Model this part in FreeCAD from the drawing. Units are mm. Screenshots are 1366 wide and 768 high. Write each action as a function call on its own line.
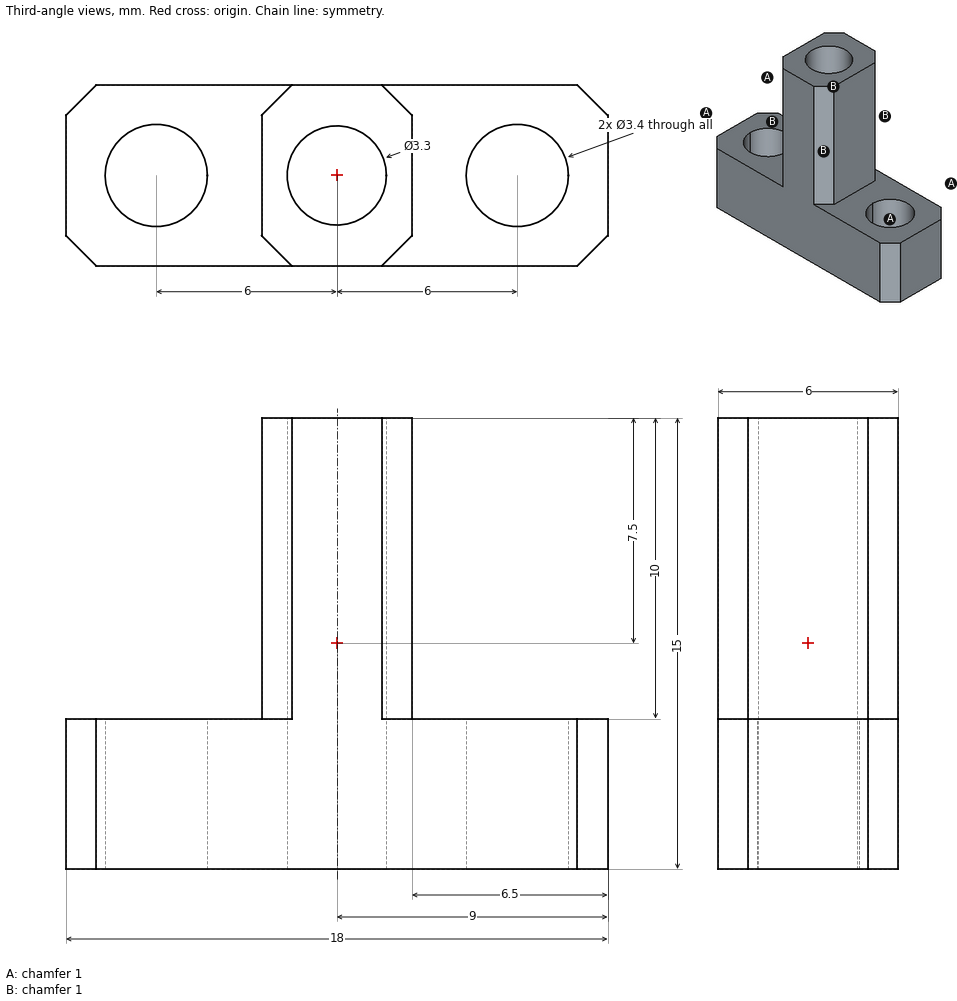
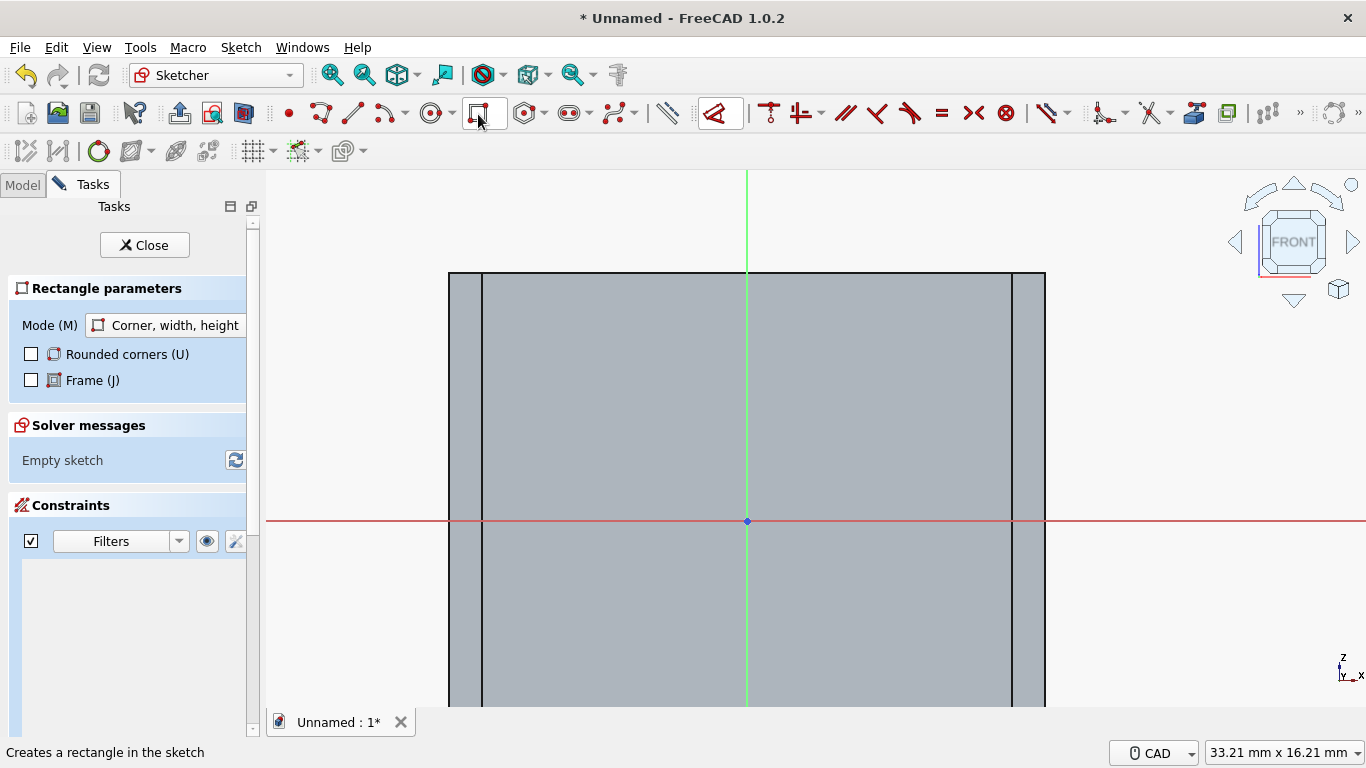
click(830, 273)
click(1045, 604)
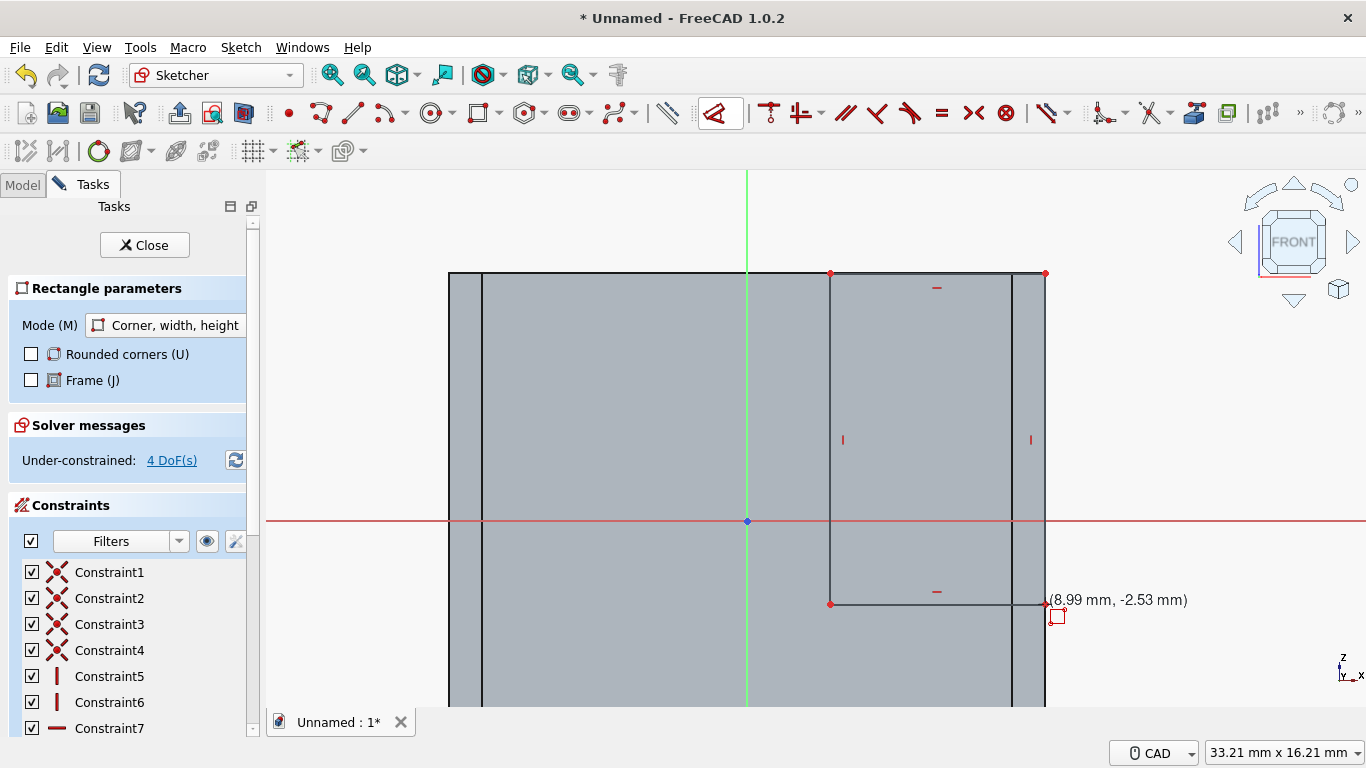
click(449, 273)
click(665, 604)
key(Escape)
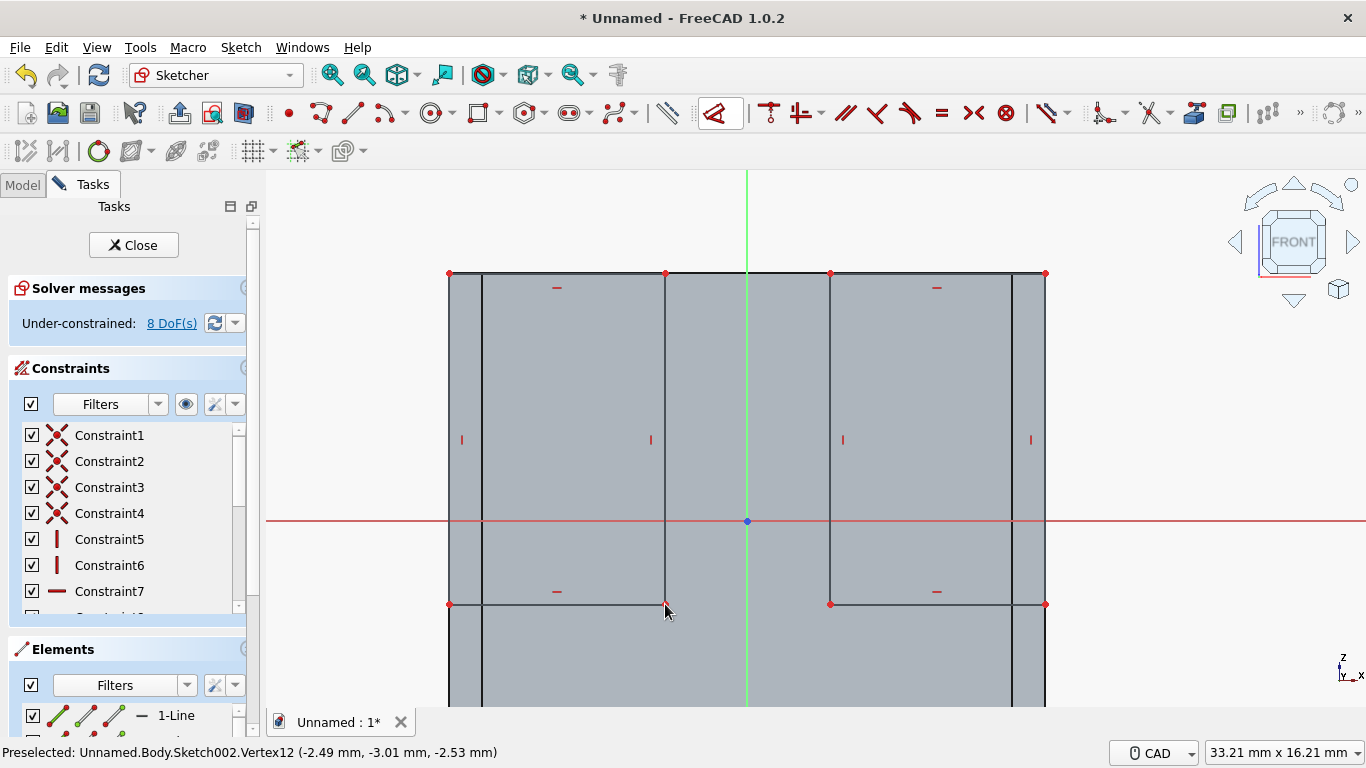
click(1045, 274)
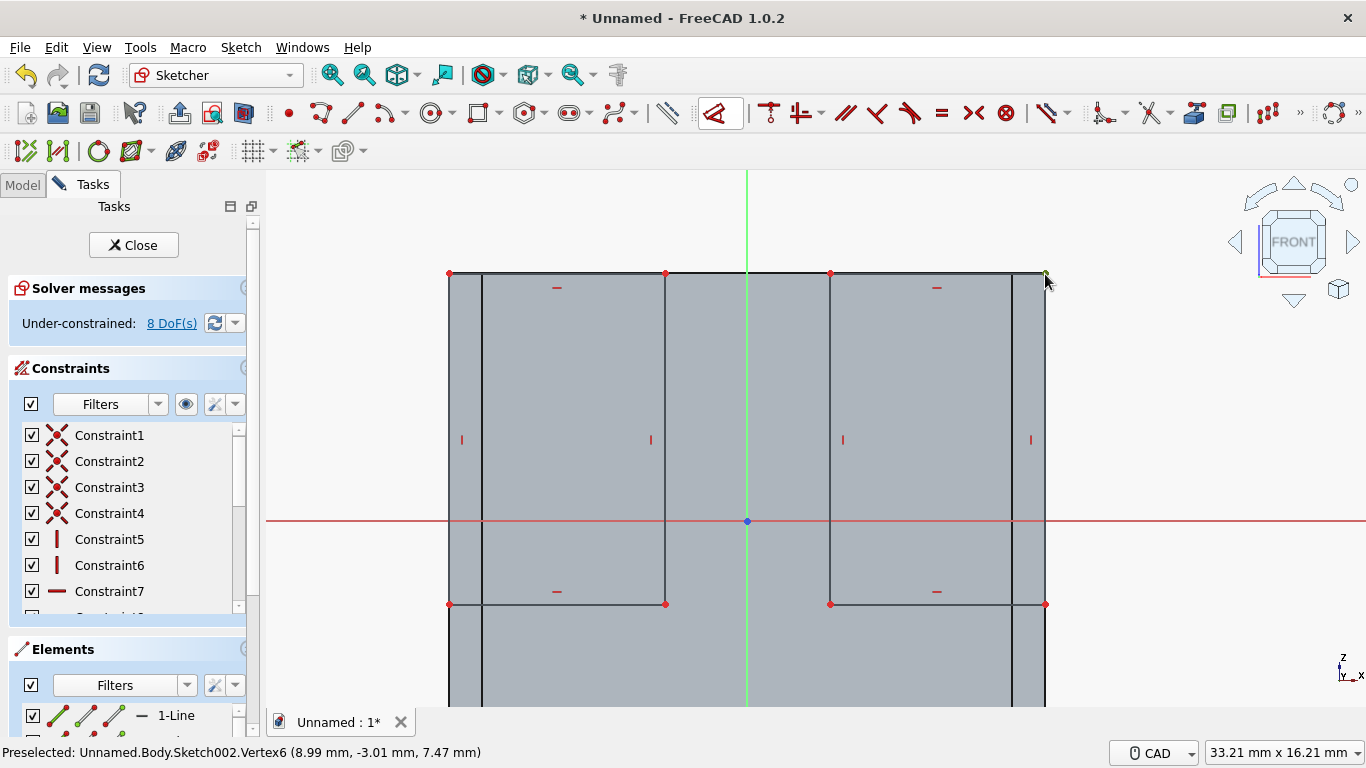
click(449, 274)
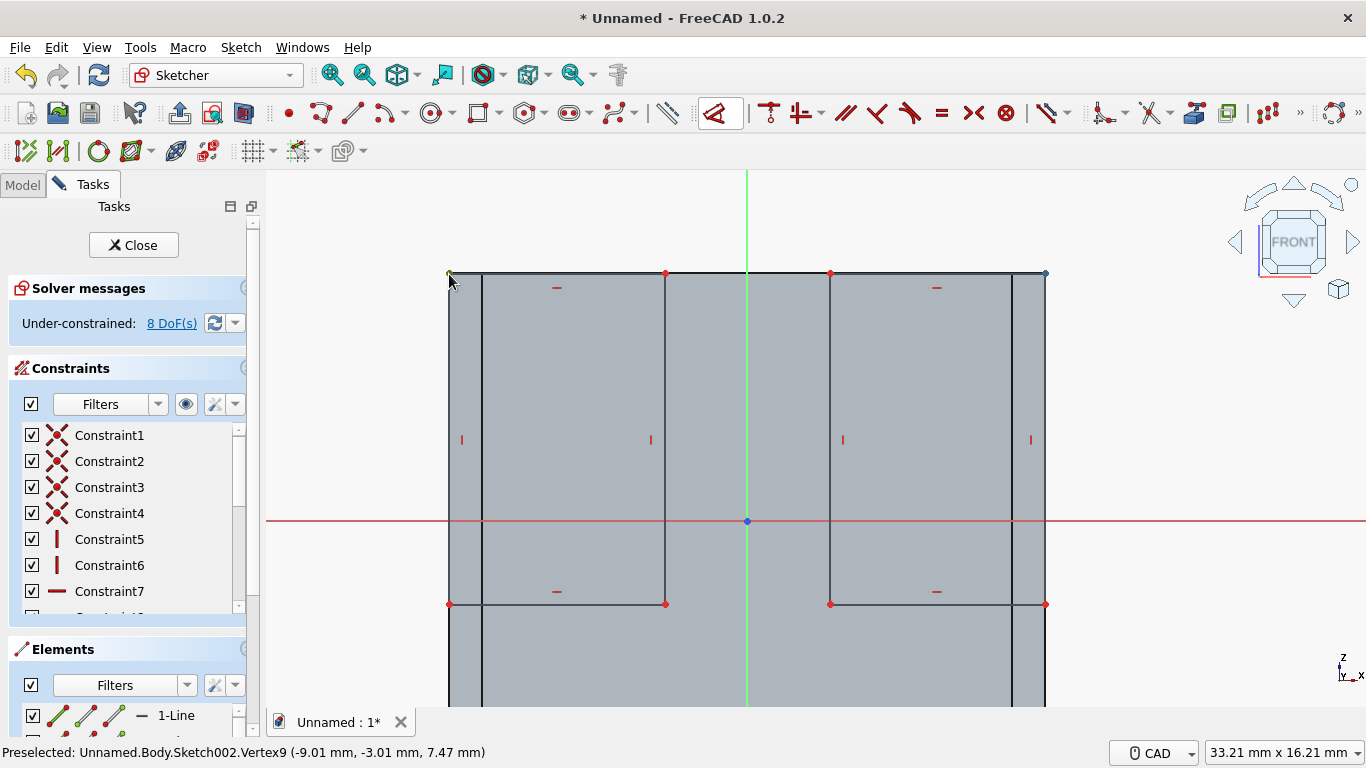
click(747, 645)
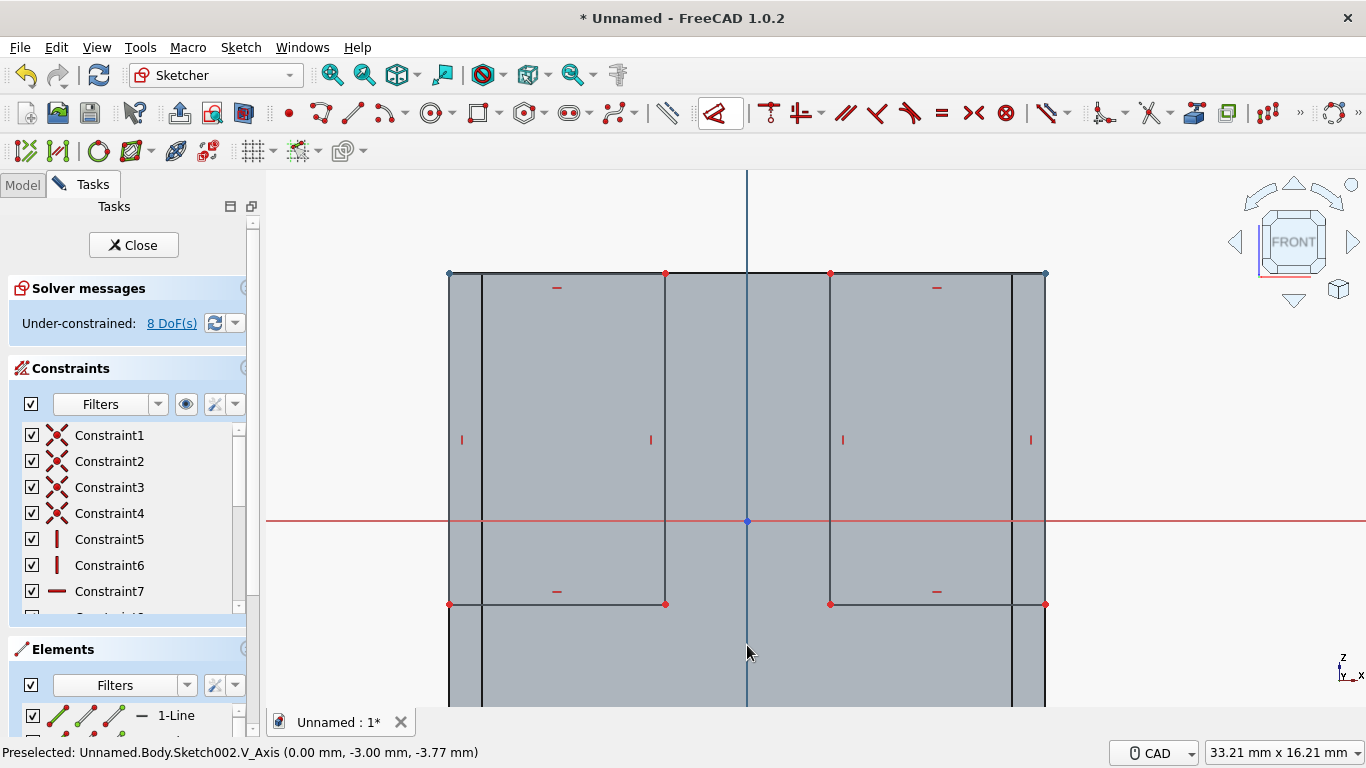
click(974, 114)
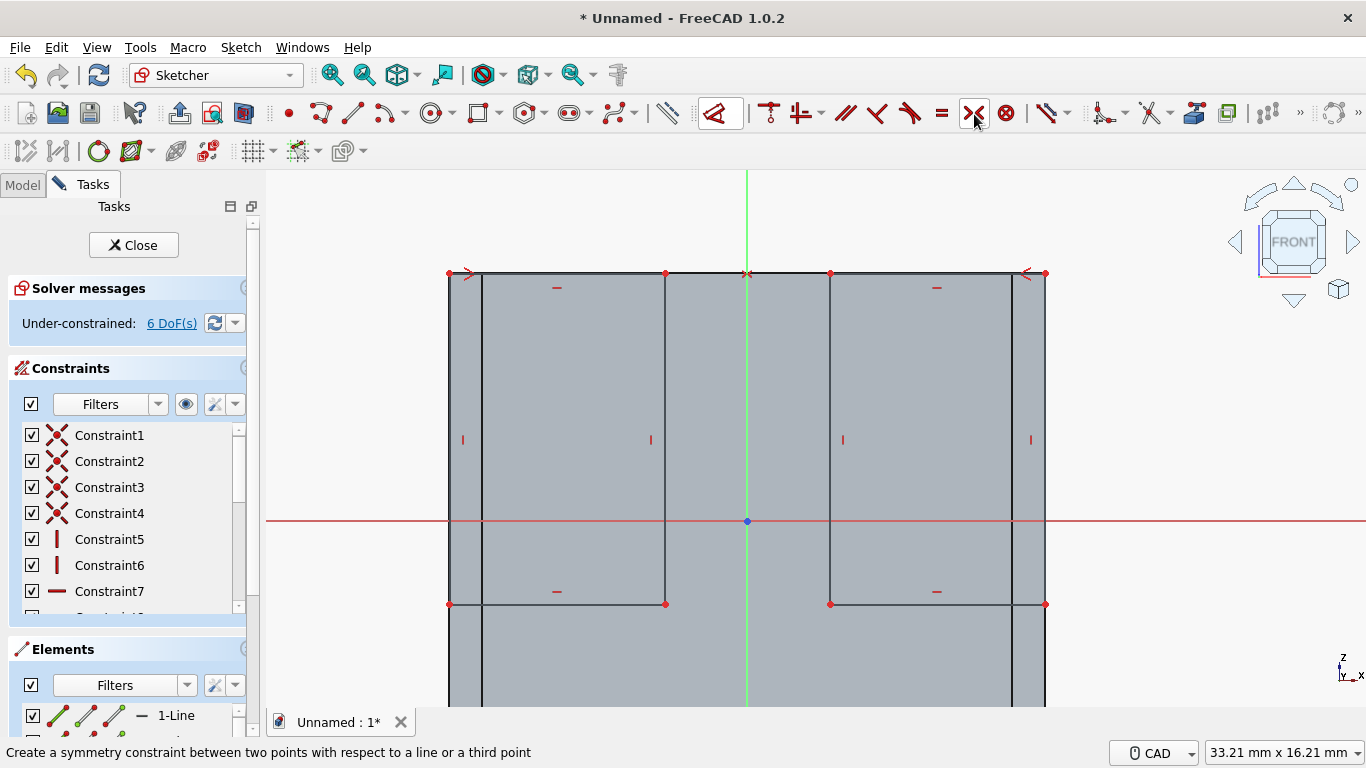
click(830, 605)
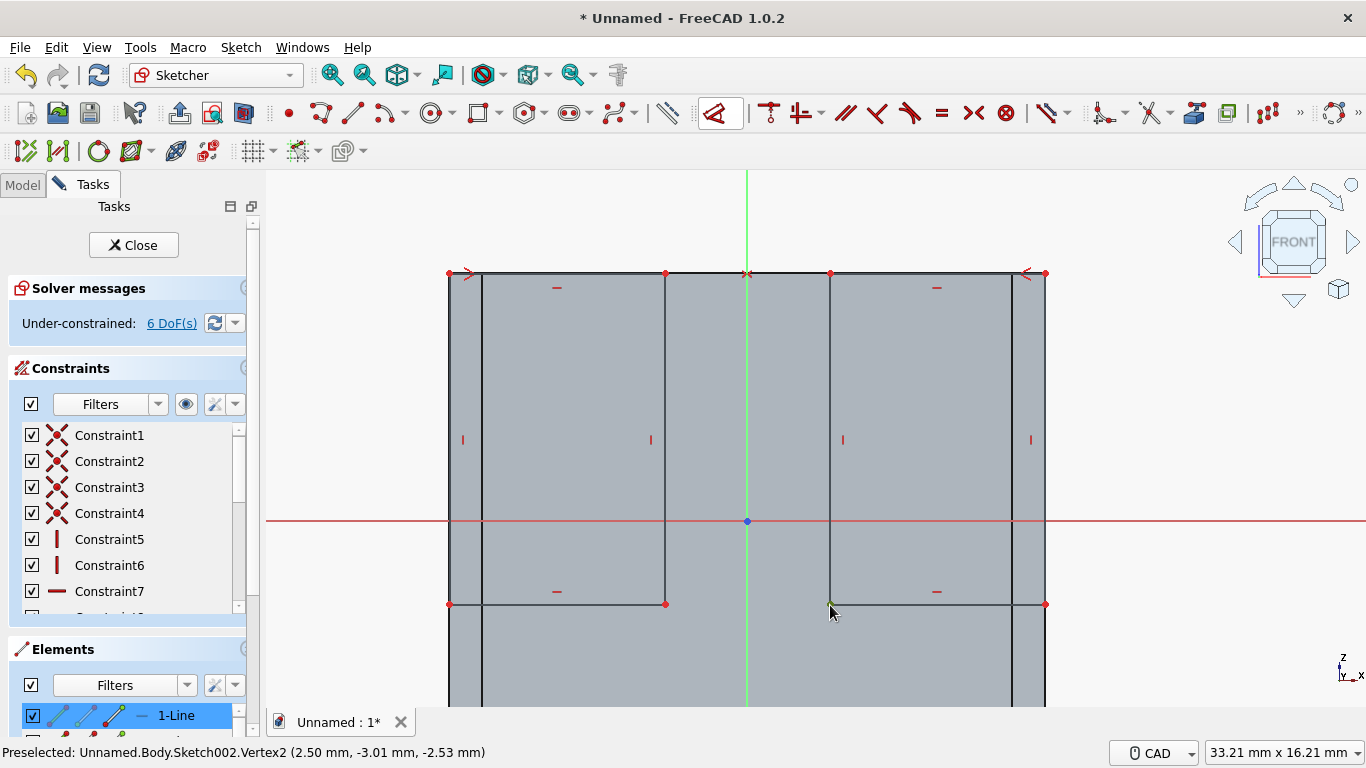
click(665, 605)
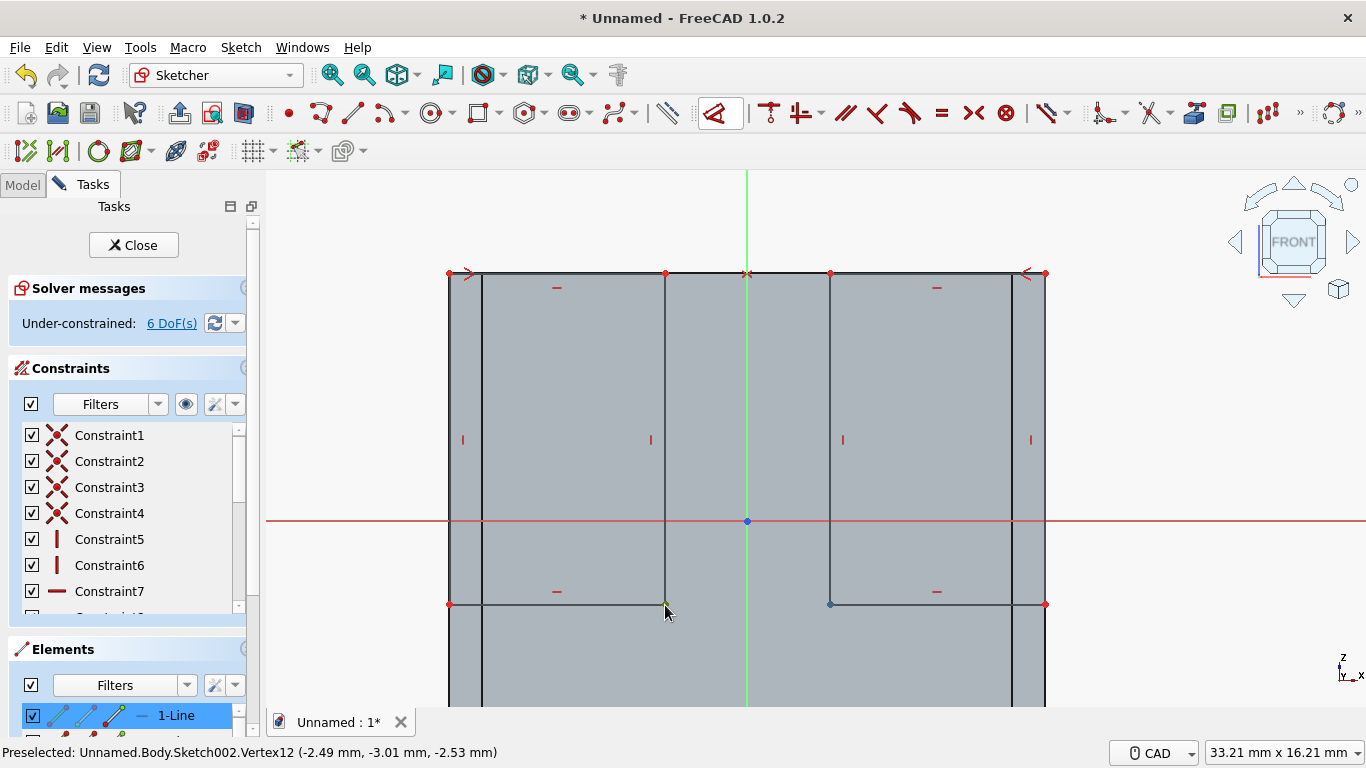
click(747, 645)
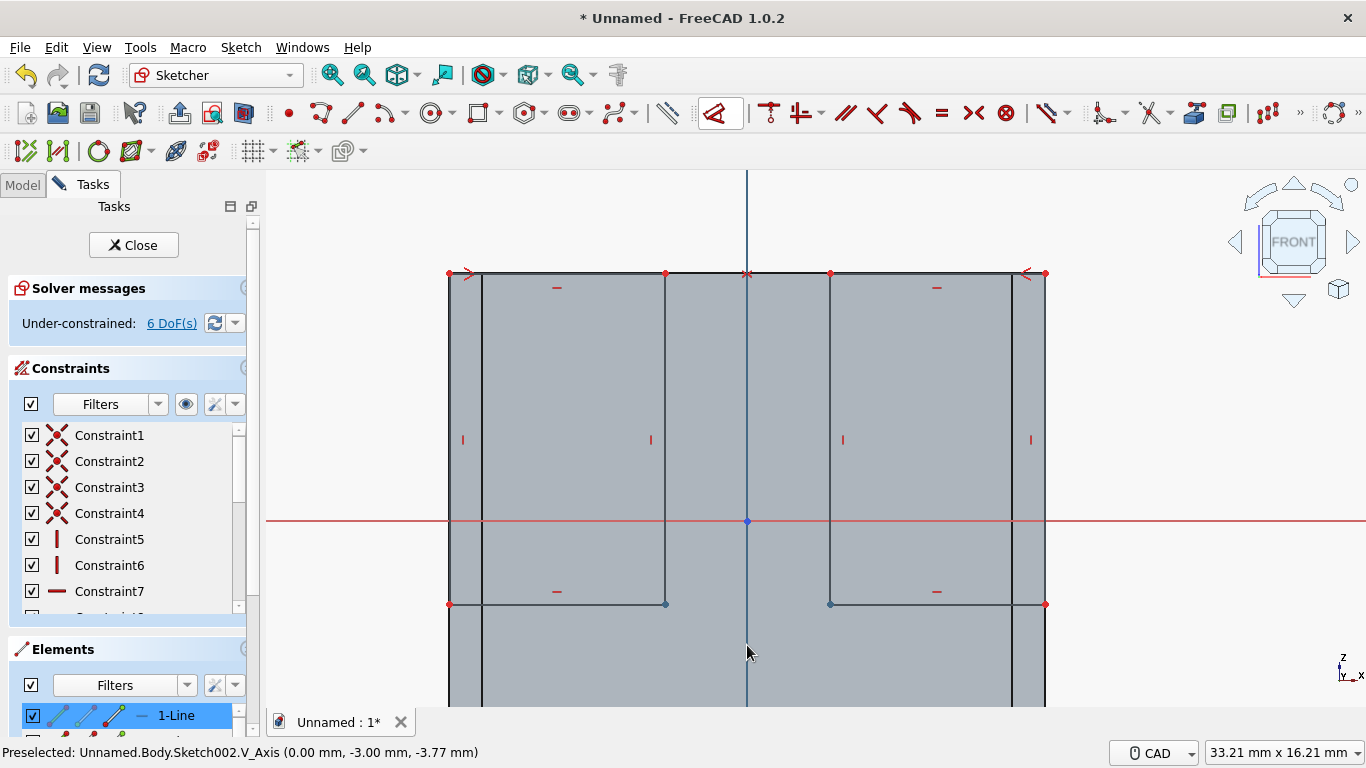
click(974, 114)